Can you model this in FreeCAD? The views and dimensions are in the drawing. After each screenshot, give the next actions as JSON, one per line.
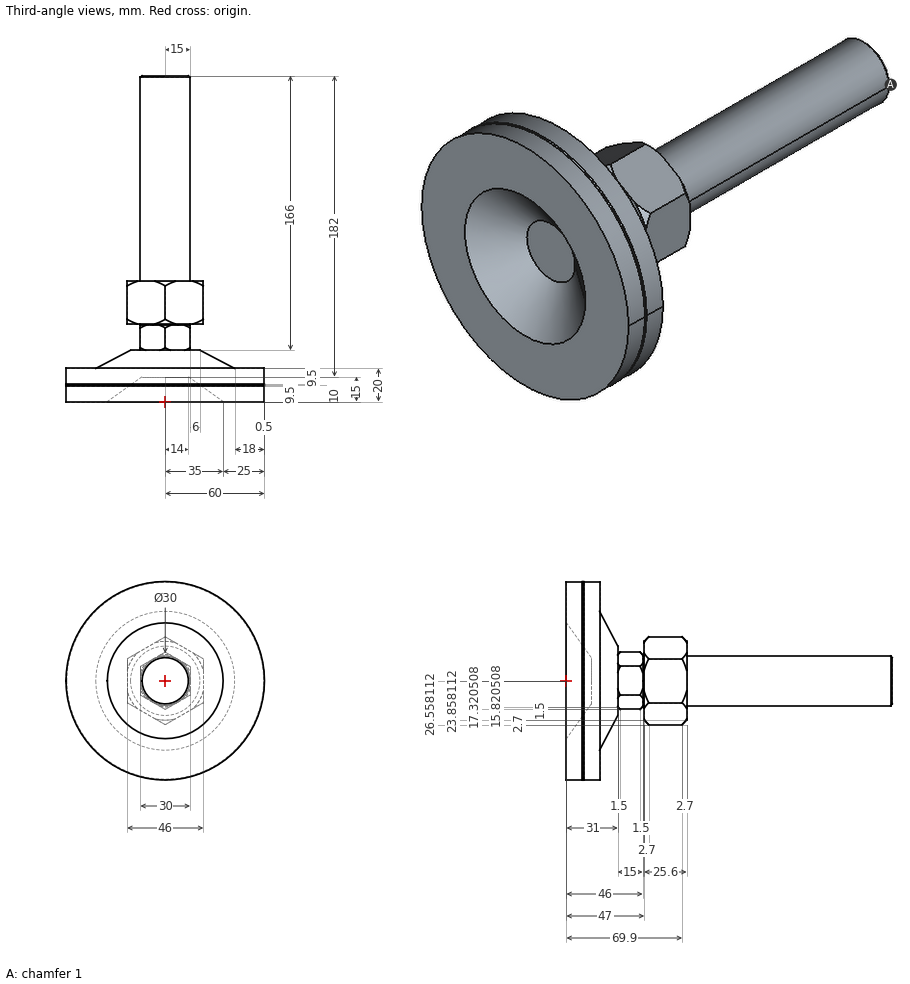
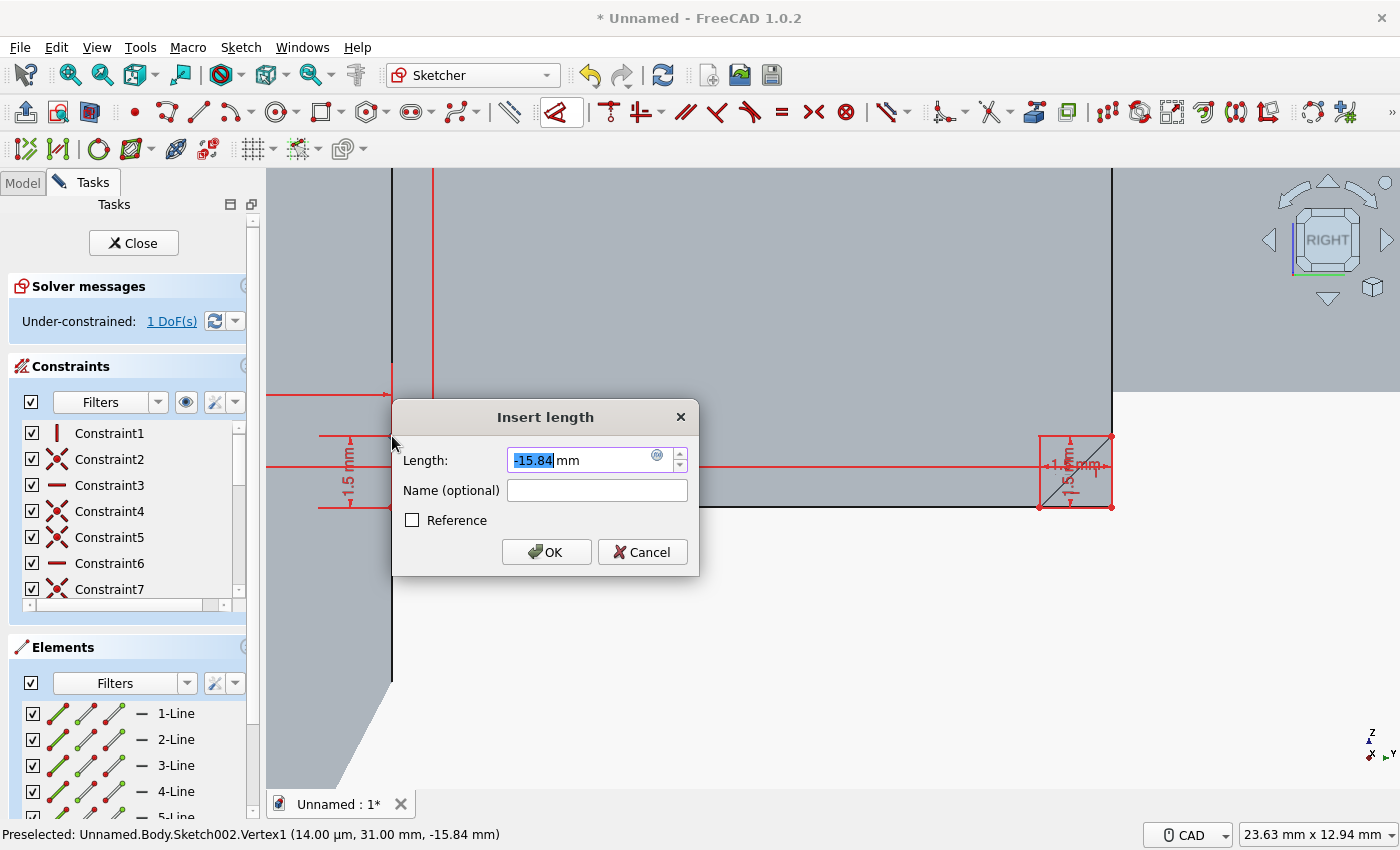
{"action": "type", "text": "-15.820508"}
{"action": "key", "text": "Return"}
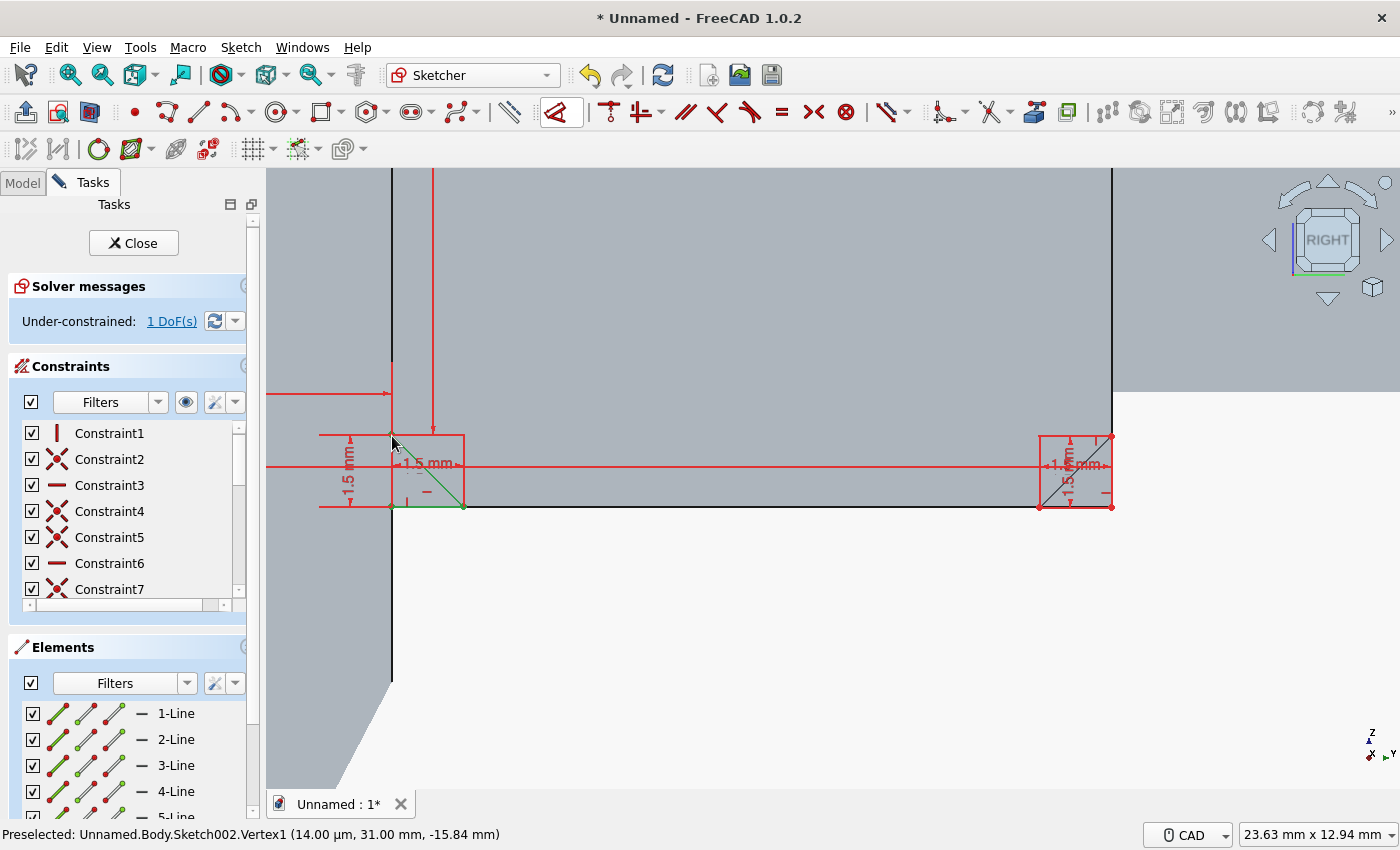
{"action": "left_click", "coordinate": [1040, 508]}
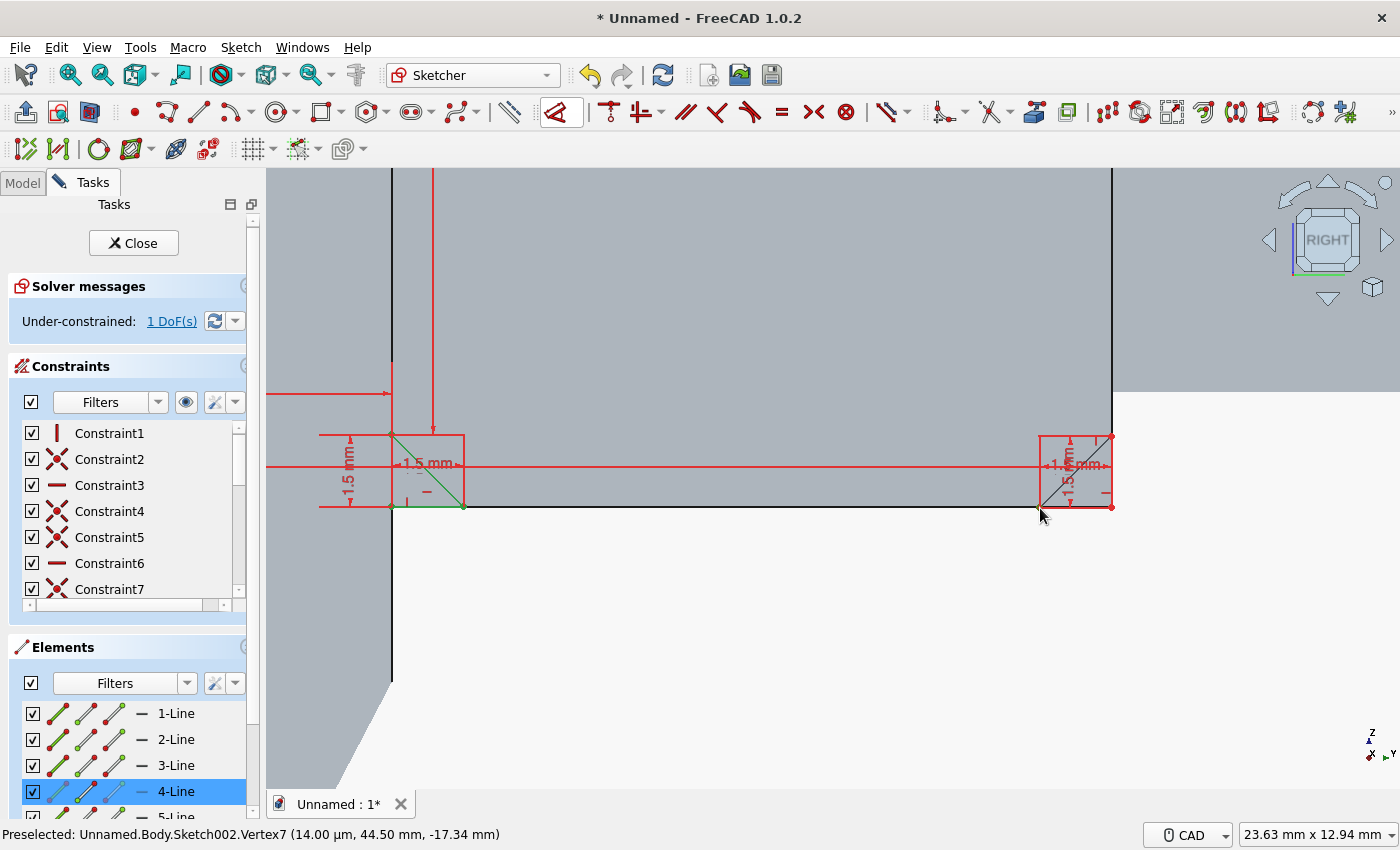
{"action": "left_click", "coordinate": [578, 112]}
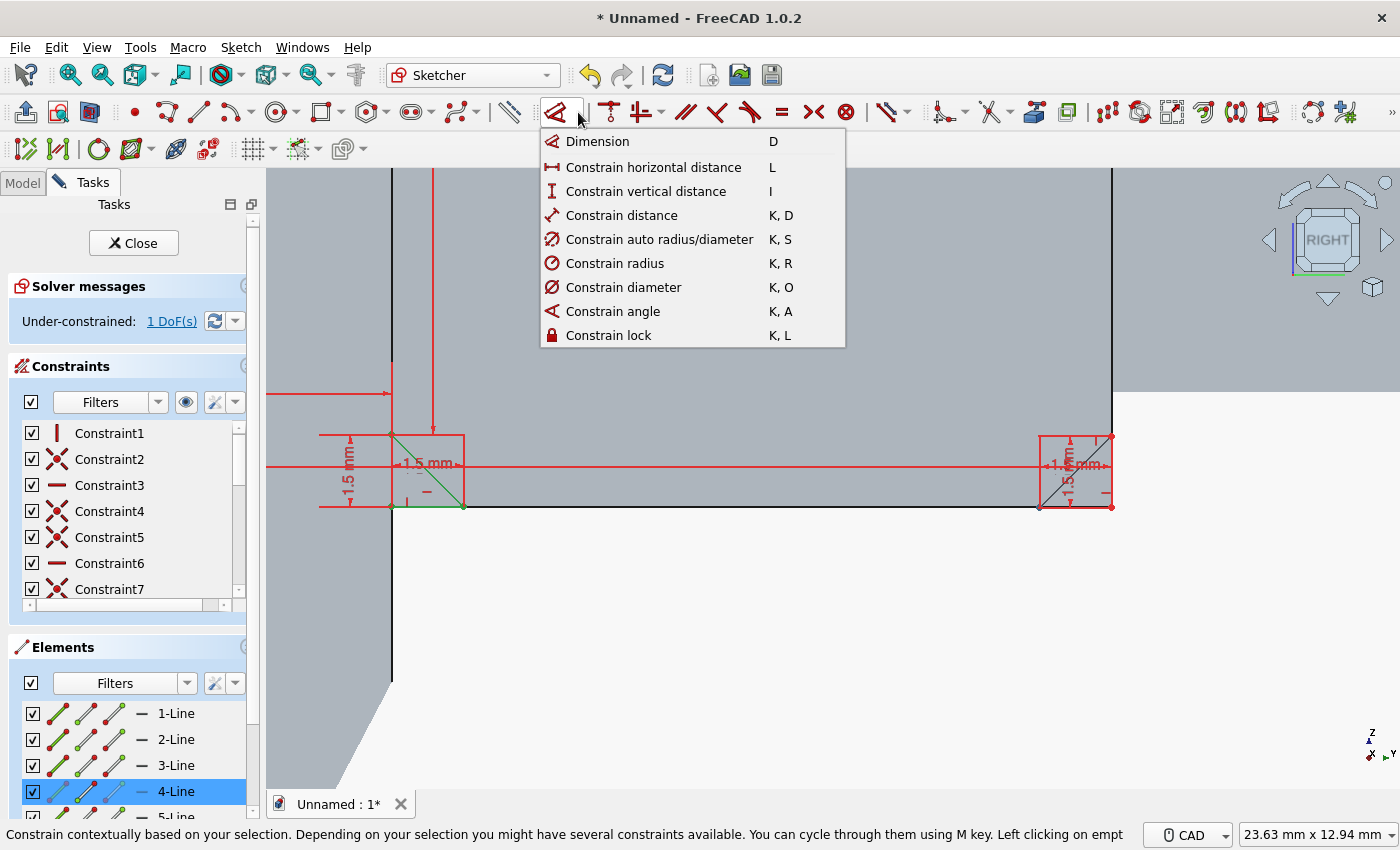
{"action": "left_click", "coordinate": [693, 191]}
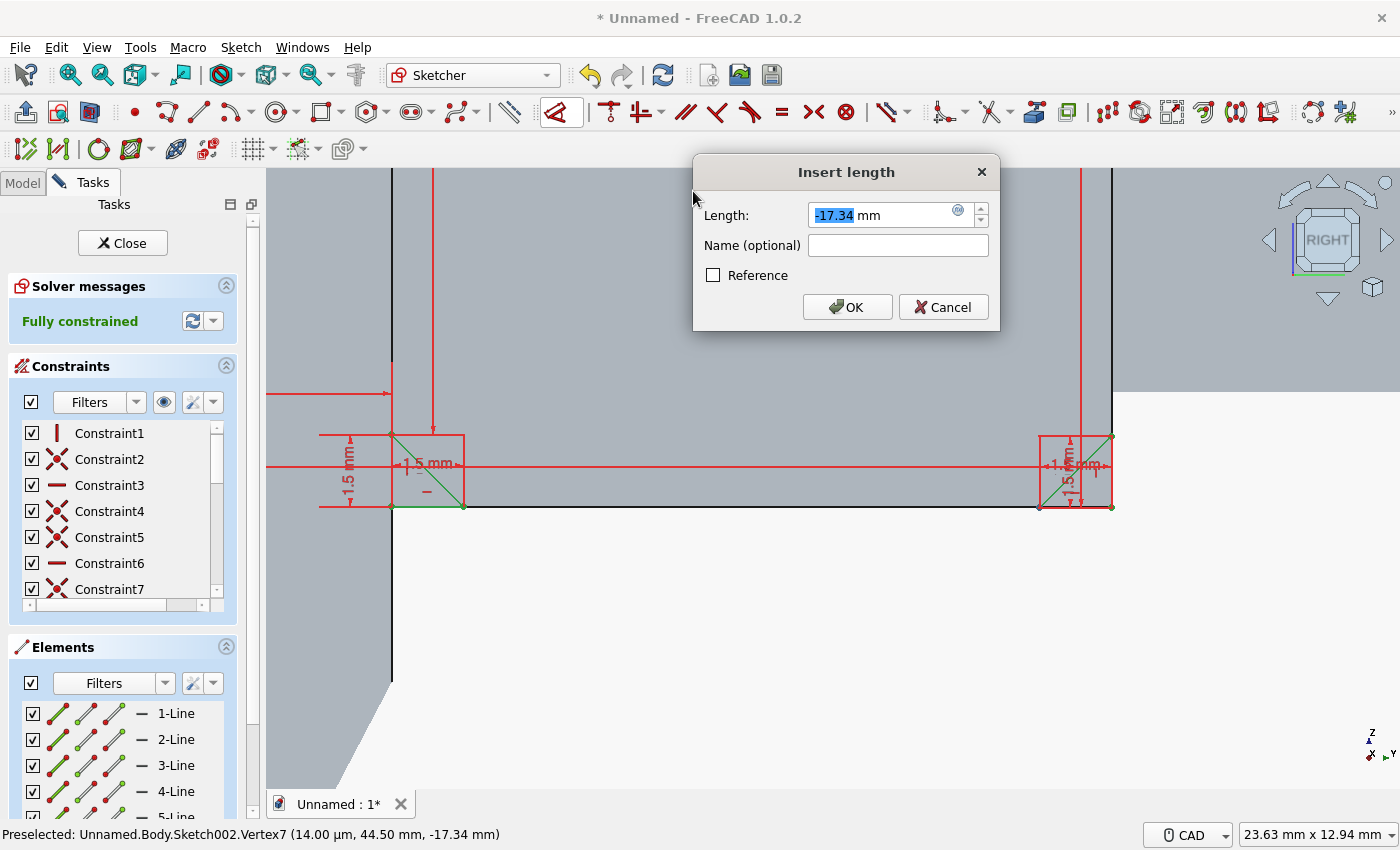
{"action": "type", "text": "-17.320508"}
{"action": "key", "text": "Return"}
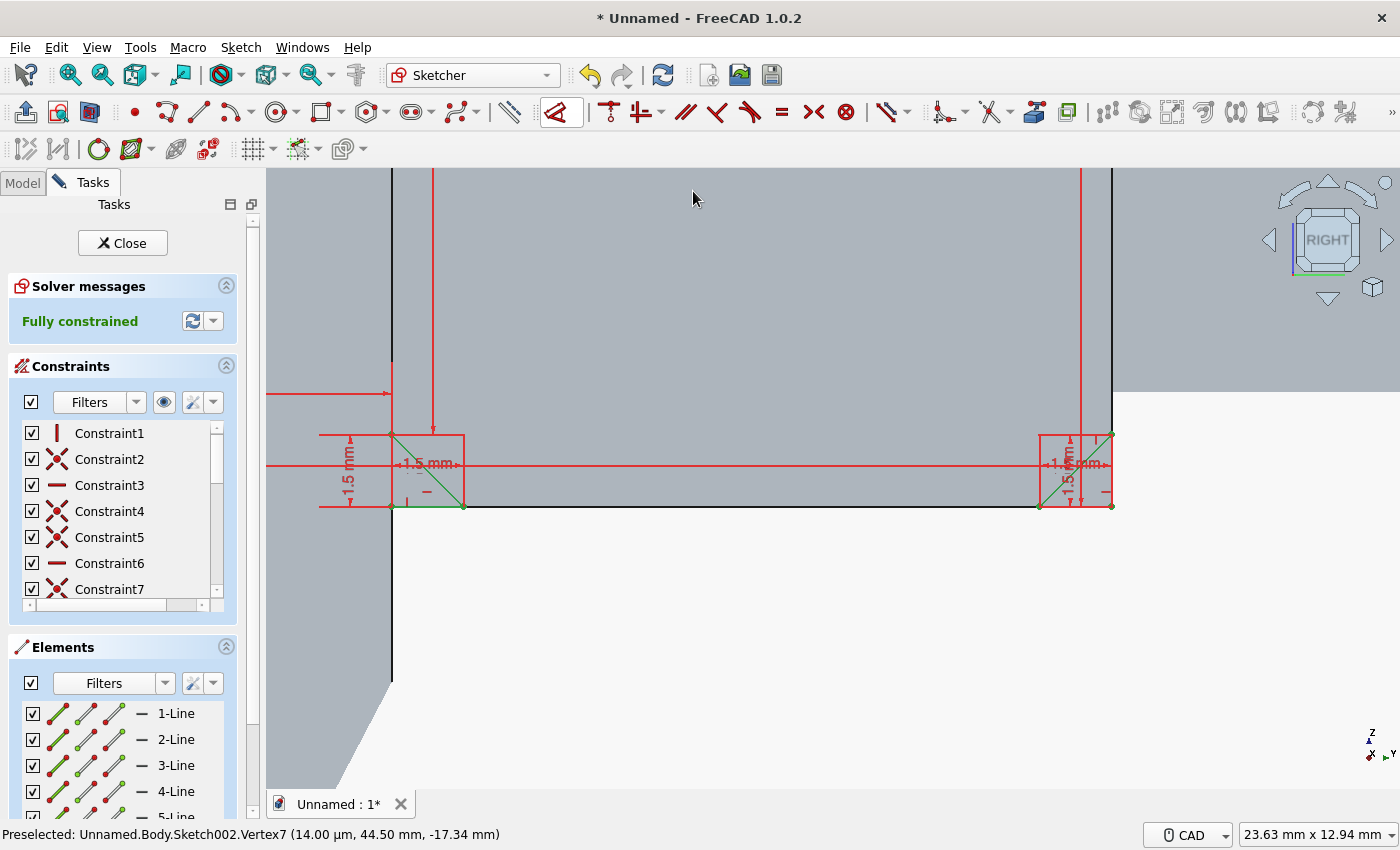
{"action": "left_click", "coordinate": [123, 243]}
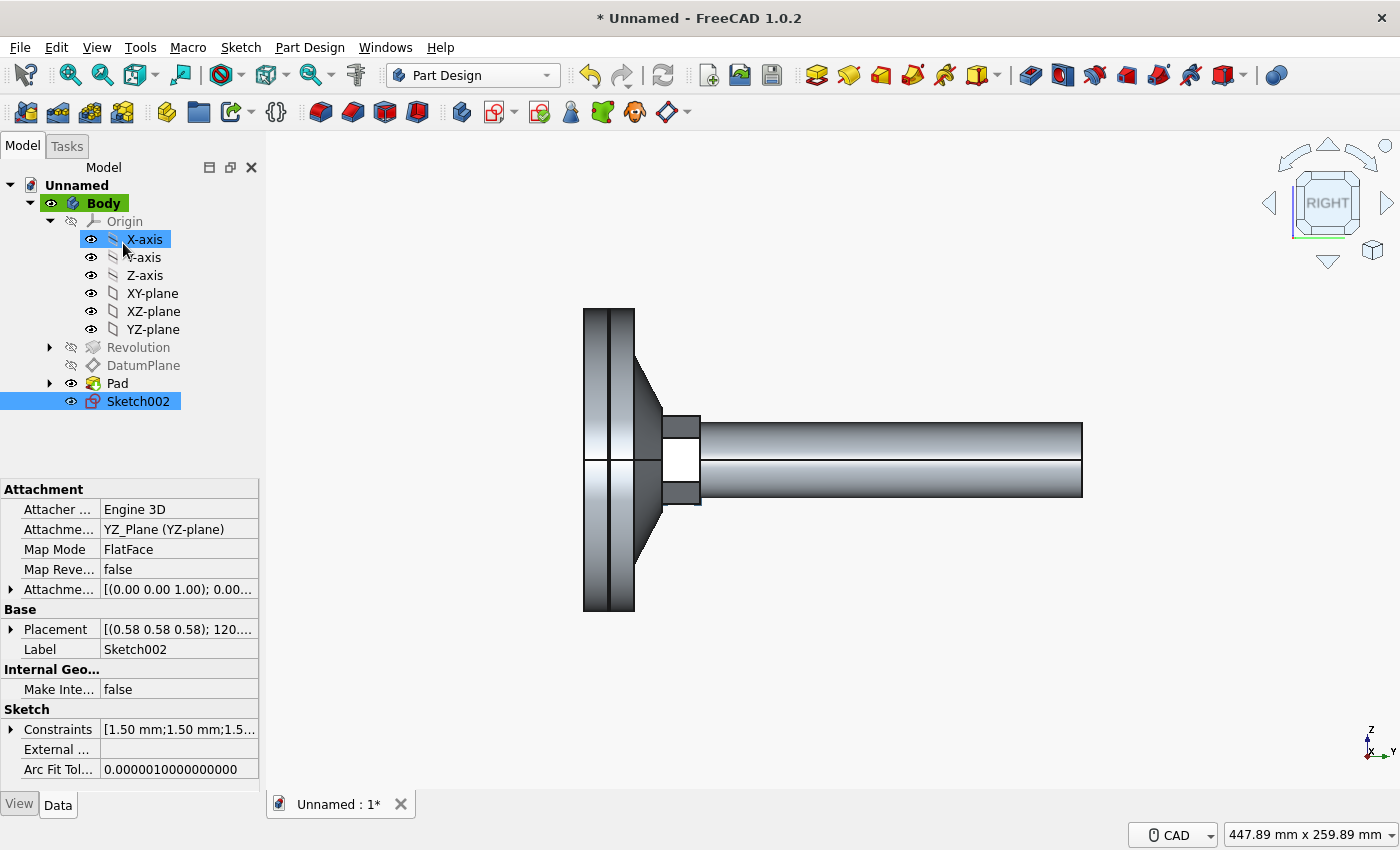
{"action": "left_click", "coordinate": [1096, 76]}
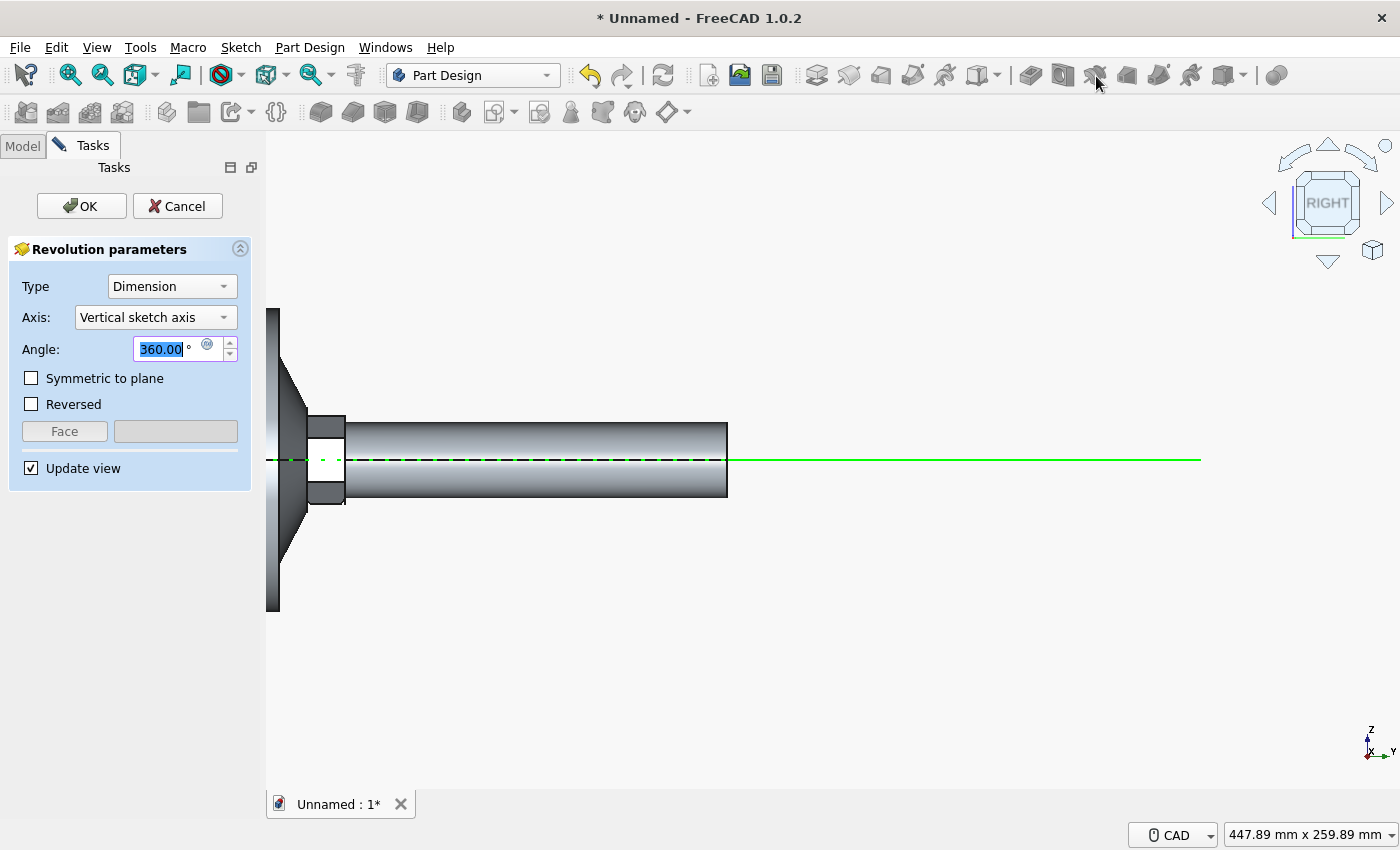
{"action": "left_click", "coordinate": [156, 318]}